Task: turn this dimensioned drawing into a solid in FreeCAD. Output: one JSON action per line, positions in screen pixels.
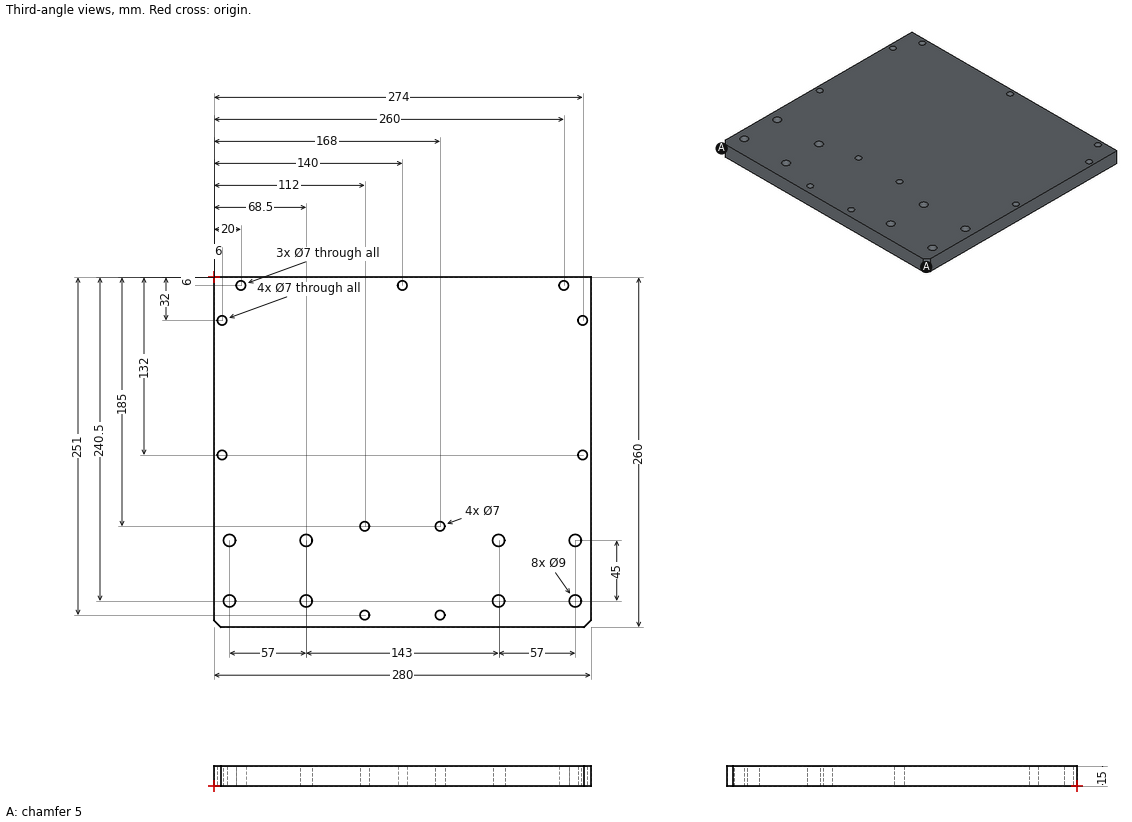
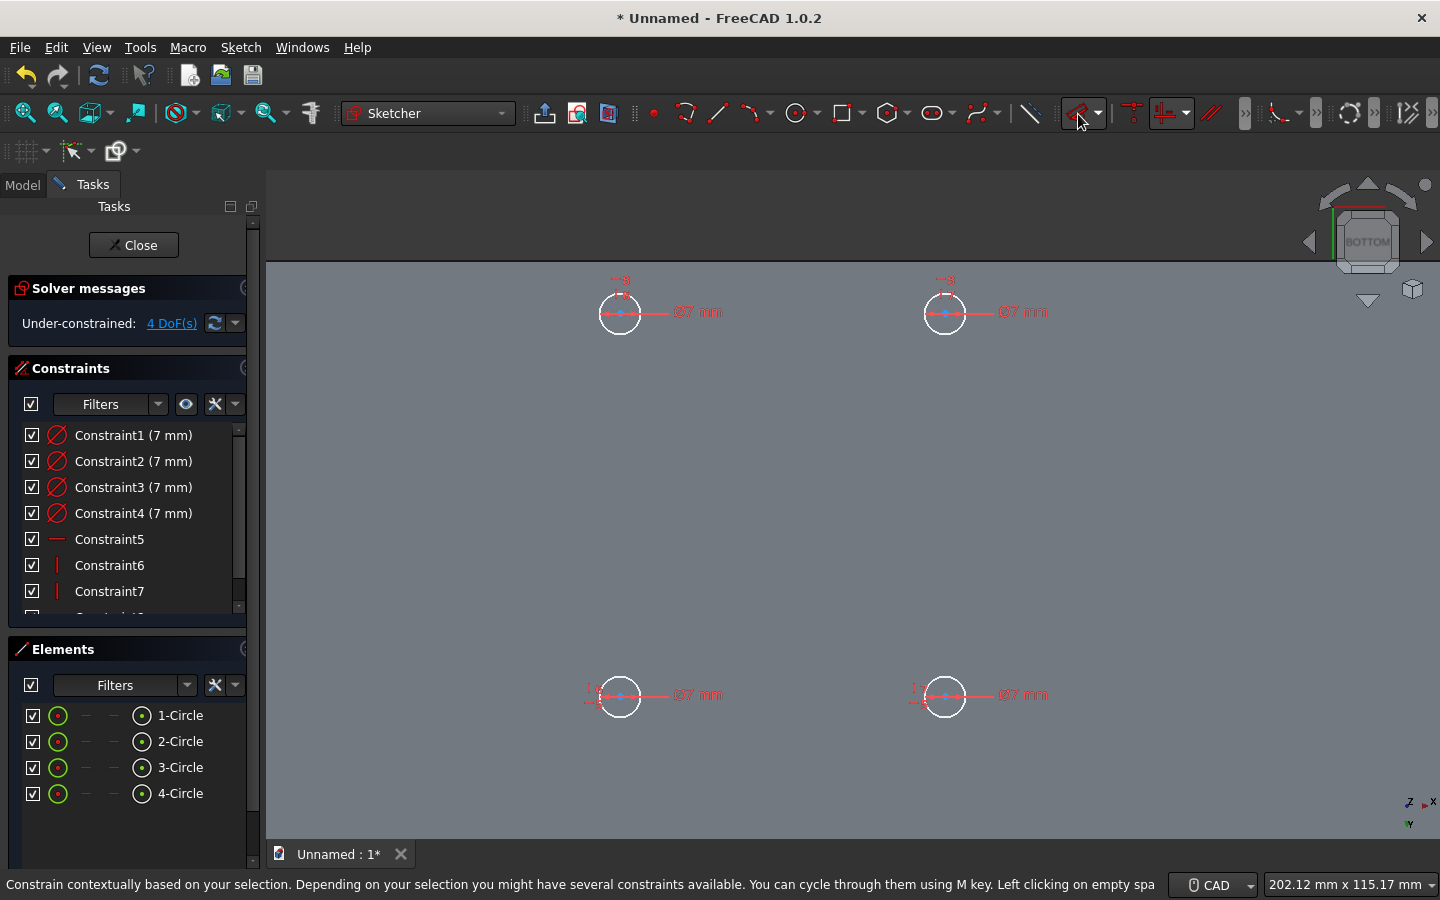
{"action": "left_click", "coordinate": [945, 697]}
{"action": "left_click", "coordinate": [619, 663]}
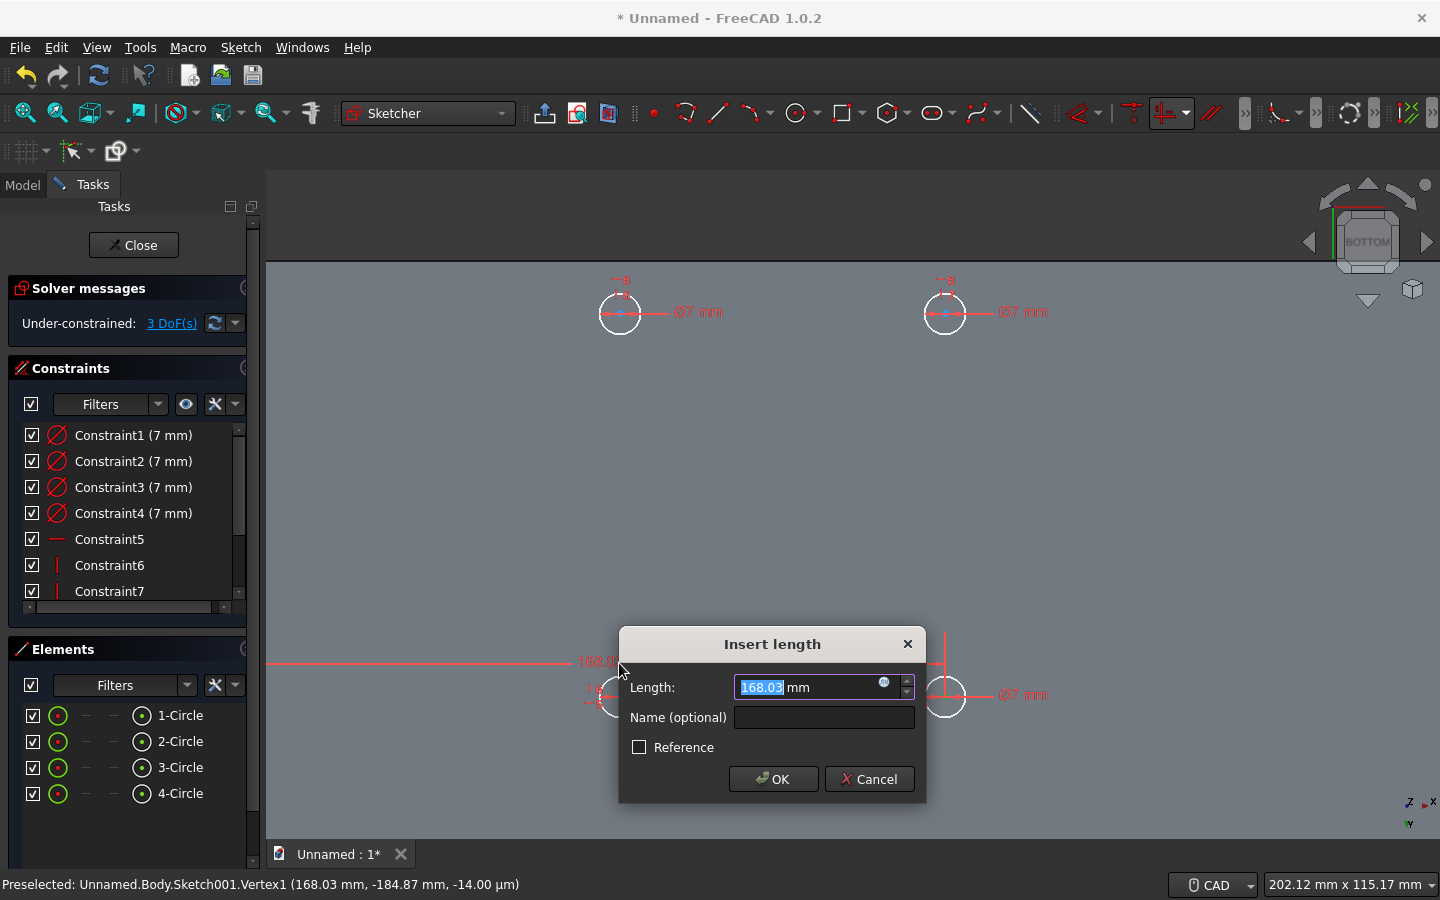
{"action": "type", "text": "168"}
{"action": "key", "text": "Return"}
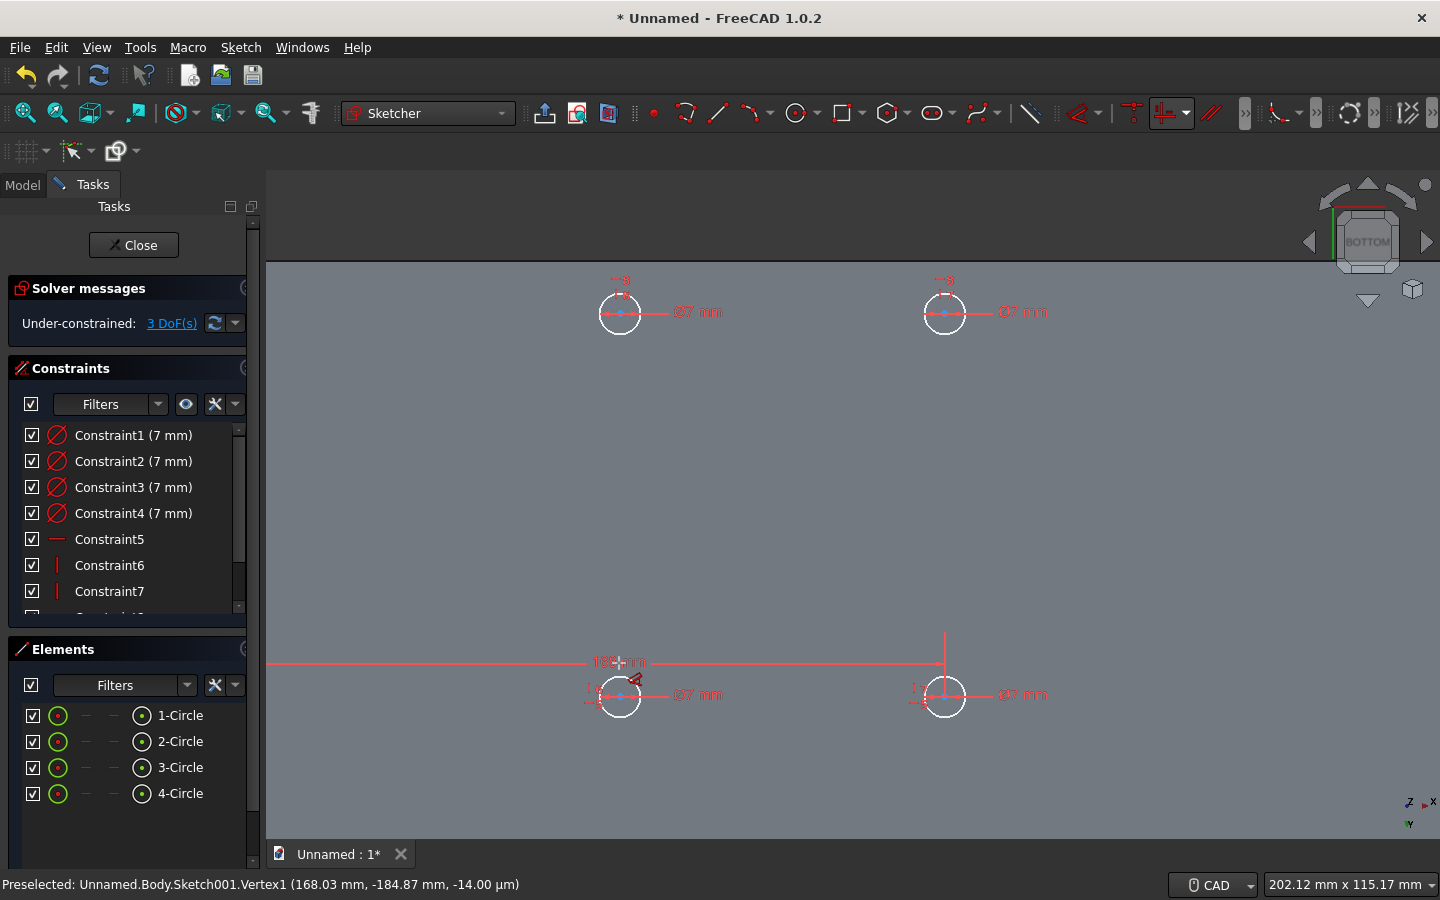
{"action": "left_click", "coordinate": [945, 697]}
{"action": "left_click", "coordinate": [979, 754]}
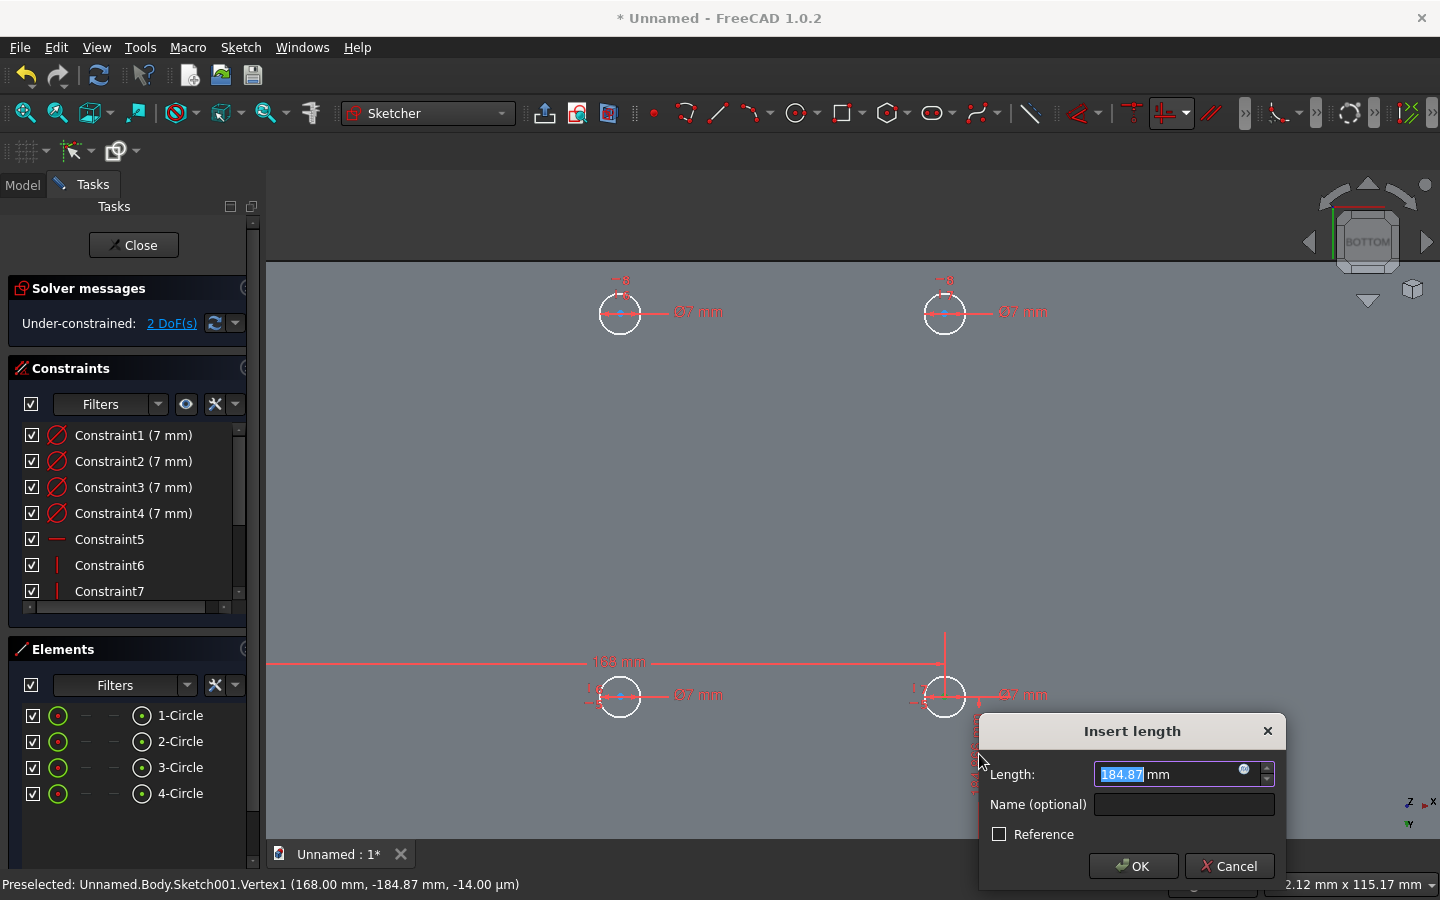
{"action": "type", "text": "185"}
{"action": "key", "text": "Return"}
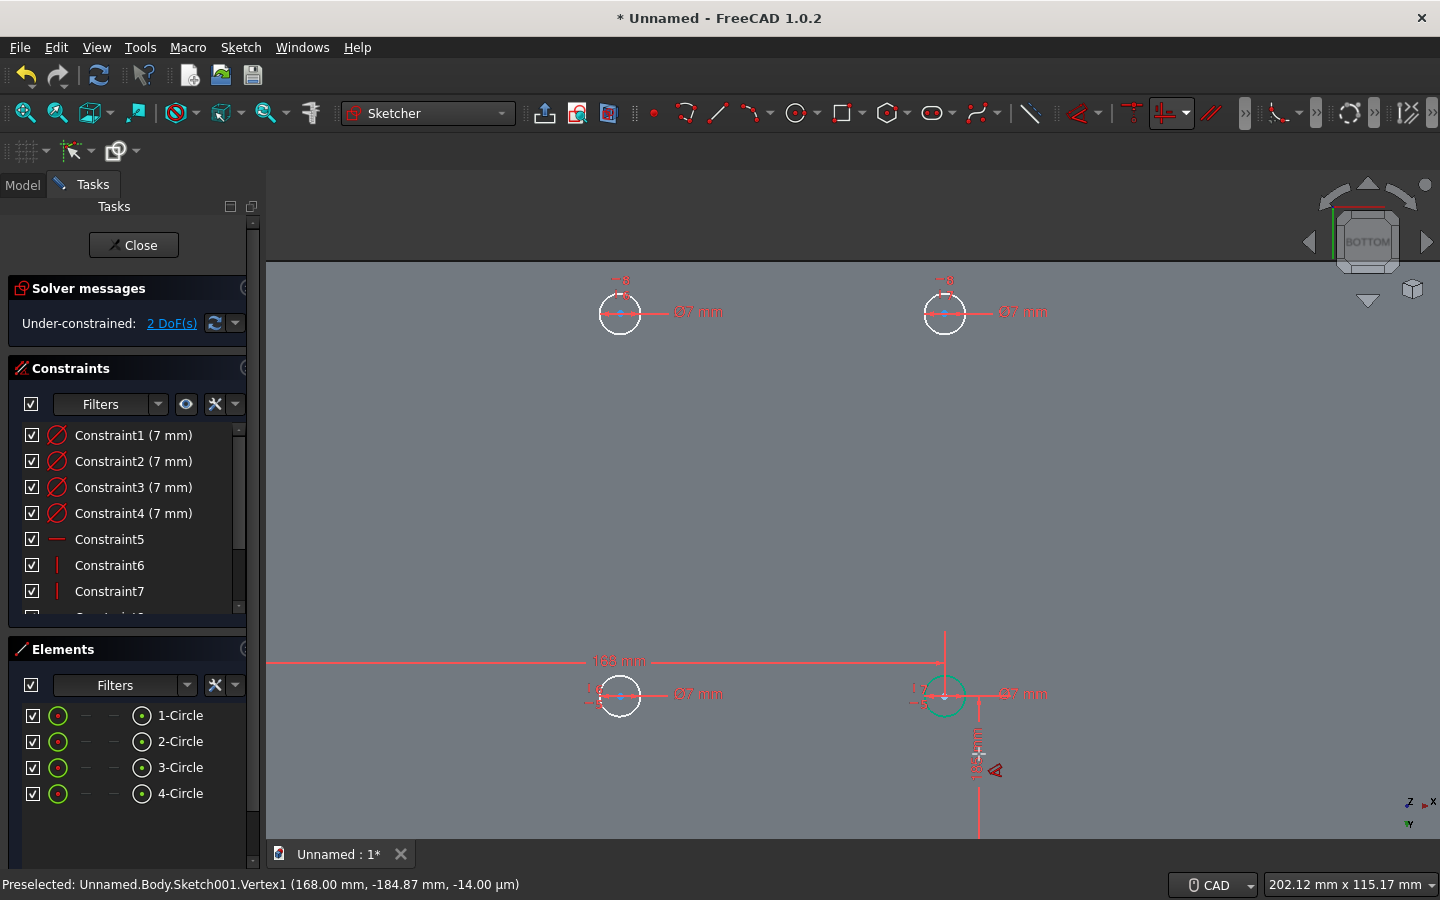
{"action": "left_click", "coordinate": [620, 696]}
{"action": "left_click", "coordinate": [457, 662]}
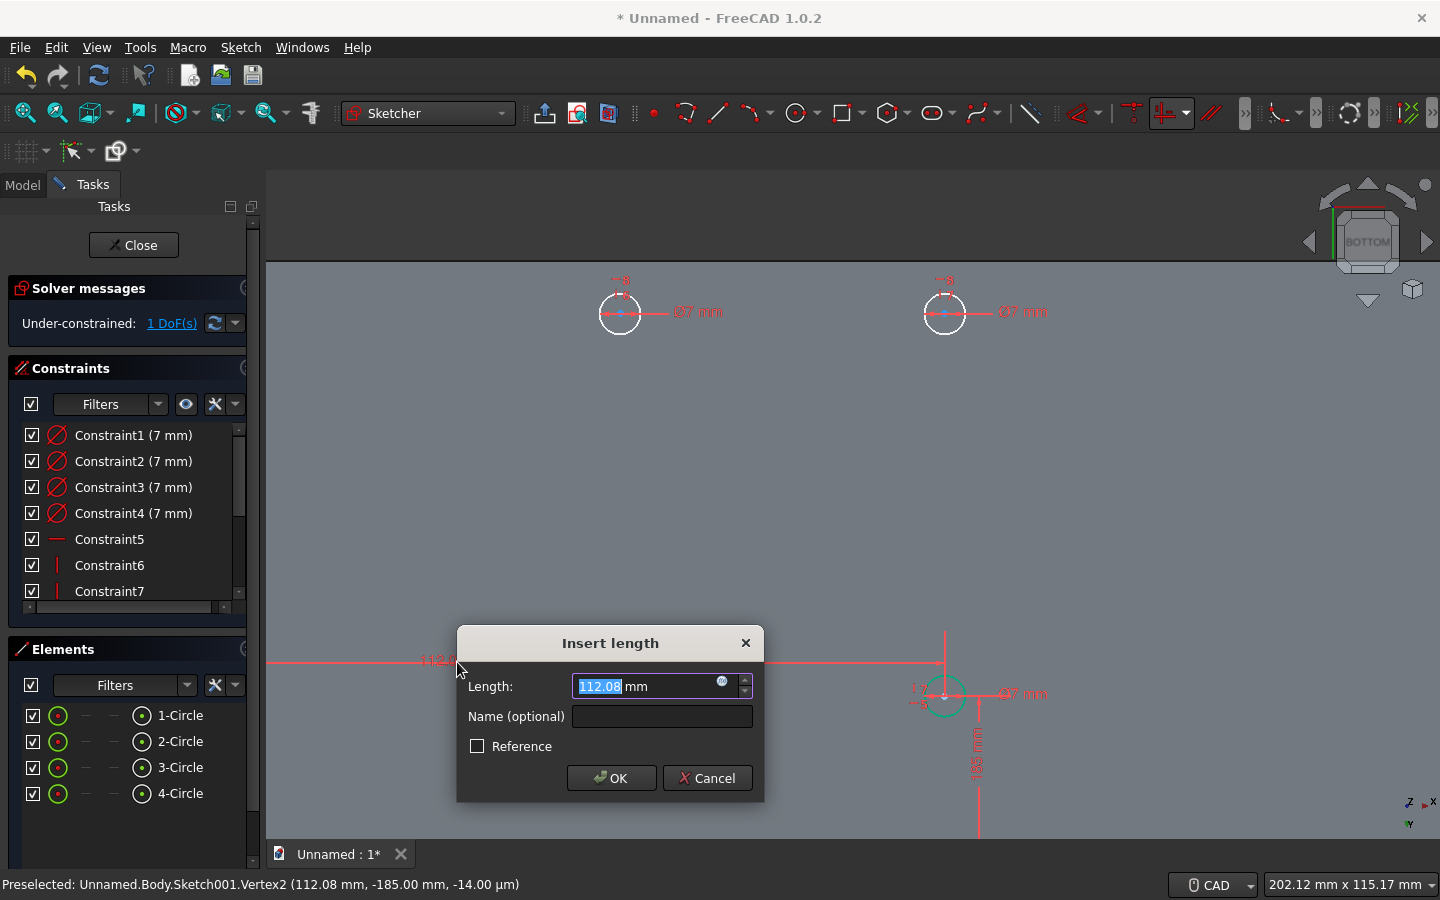
{"action": "type", "text": "112"}
{"action": "key", "text": "Return"}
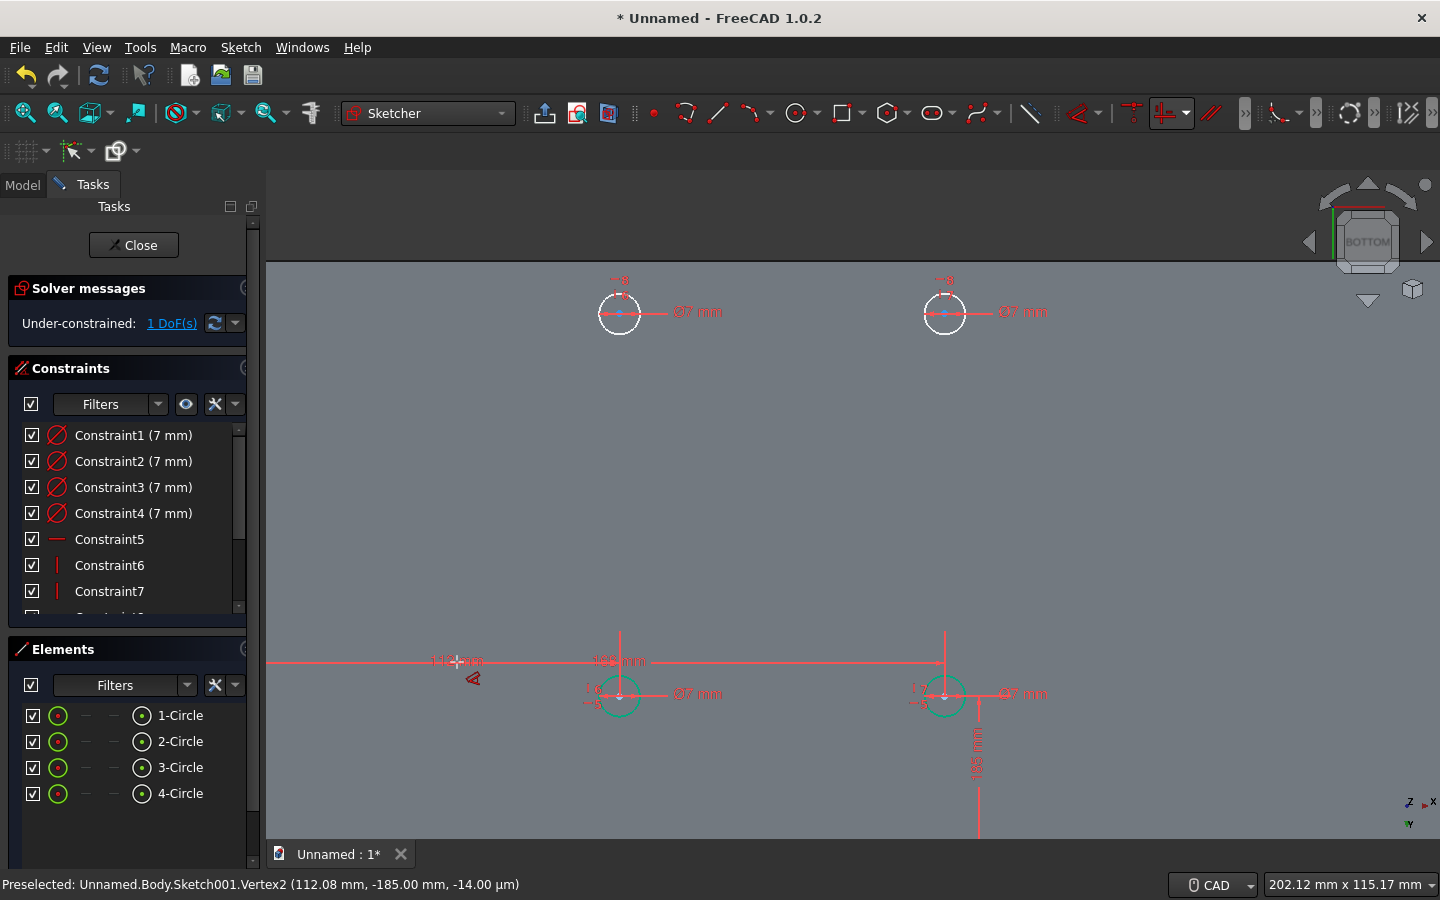
{"action": "left_click", "coordinate": [620, 314]}
{"action": "left_click", "coordinate": [654, 562]}